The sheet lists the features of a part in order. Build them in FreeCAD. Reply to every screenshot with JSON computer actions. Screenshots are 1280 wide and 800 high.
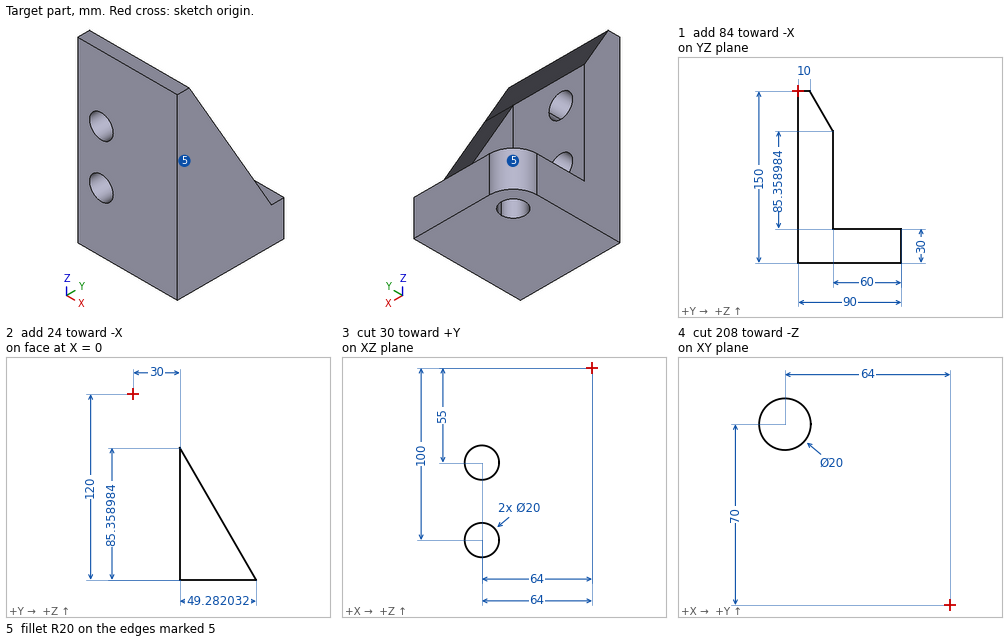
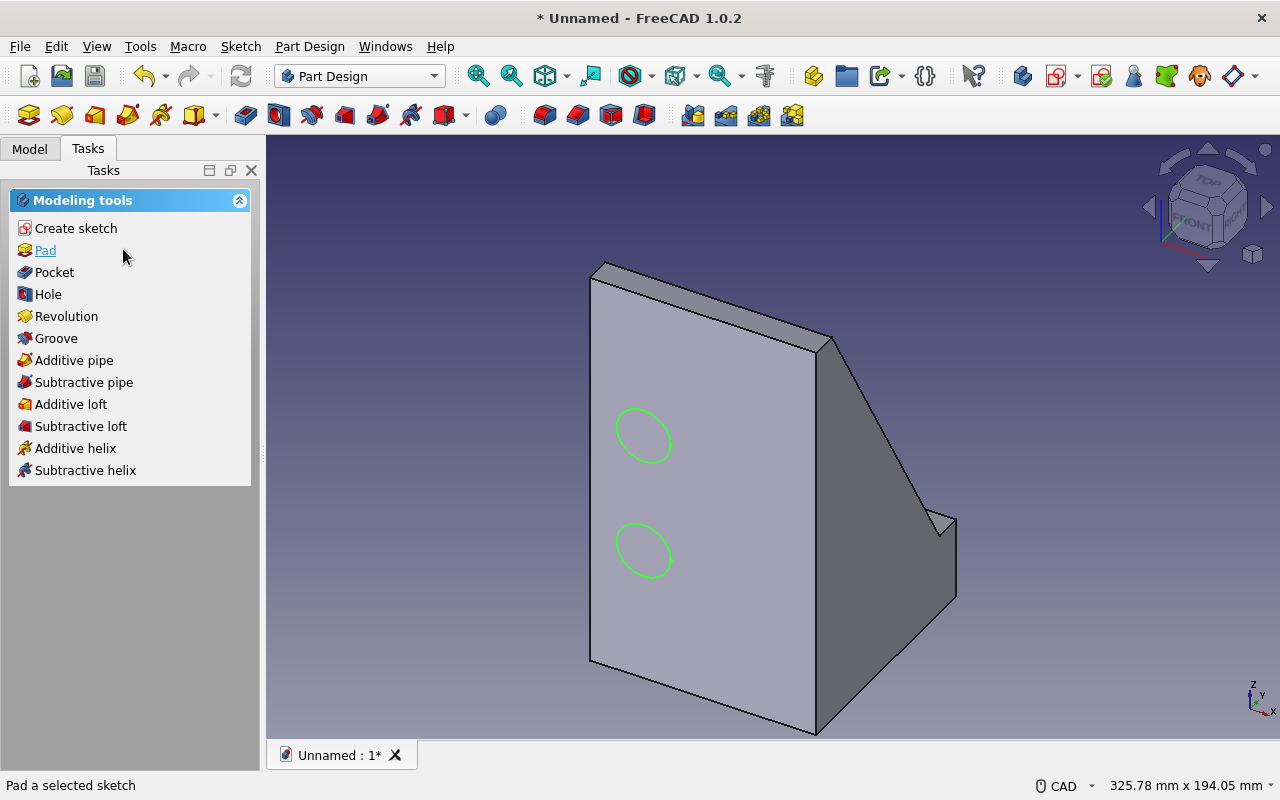
{"action": "left_click", "coordinate": [246, 116]}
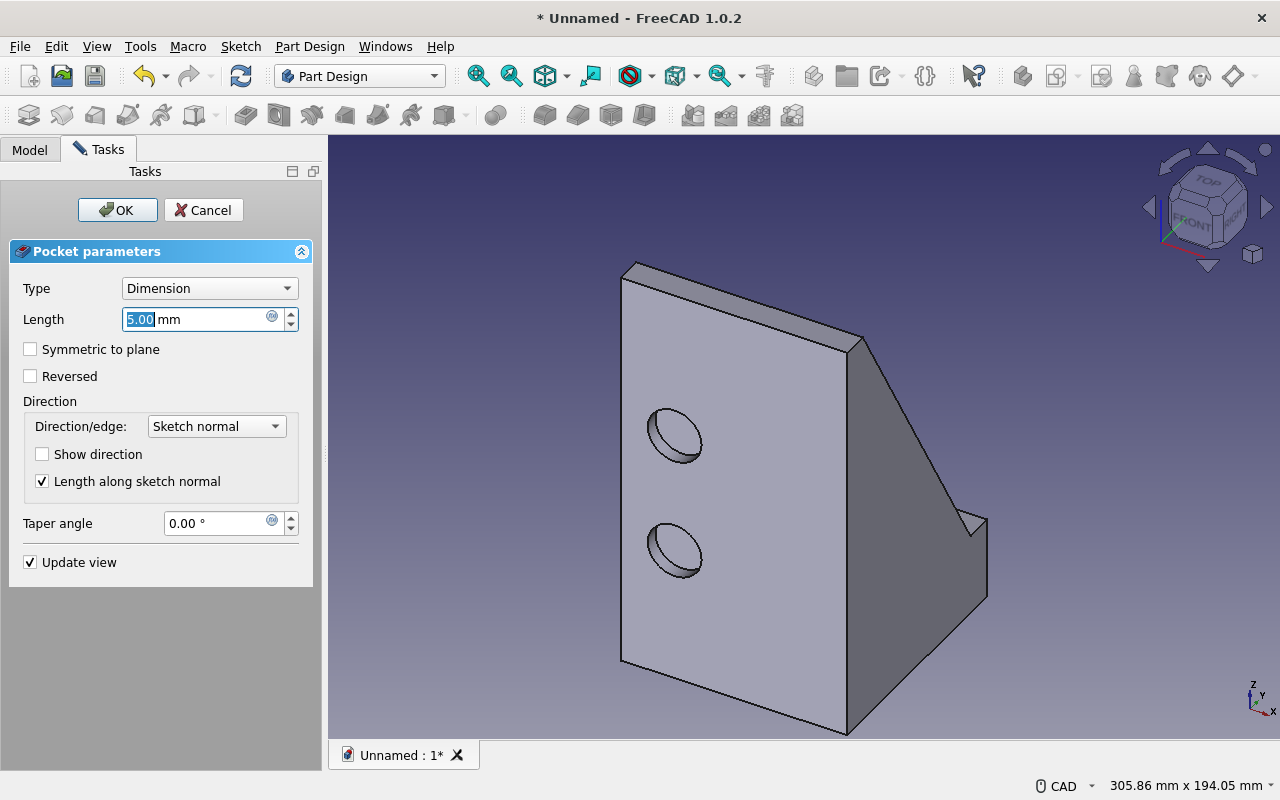
{"action": "type", "text": "30"}
{"action": "key", "text": "Tab"}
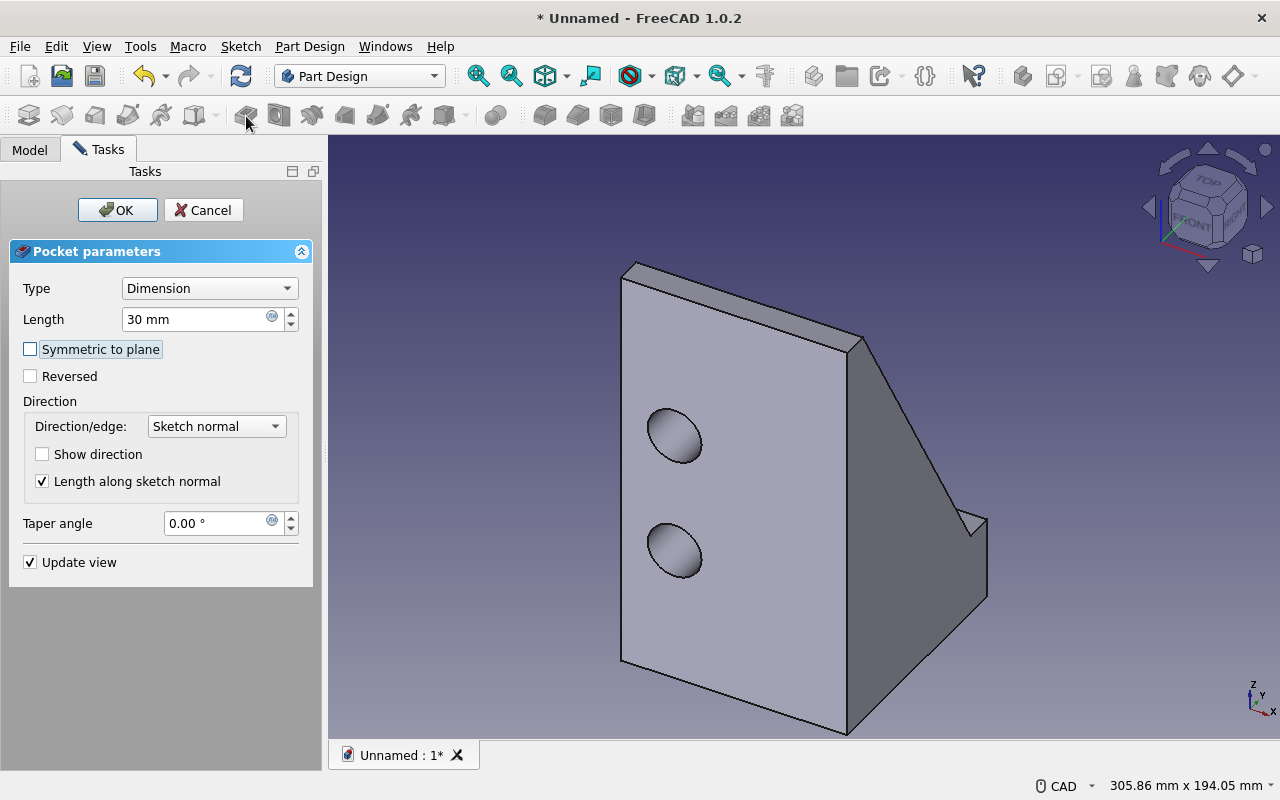
{"action": "left_click", "coordinate": [118, 210]}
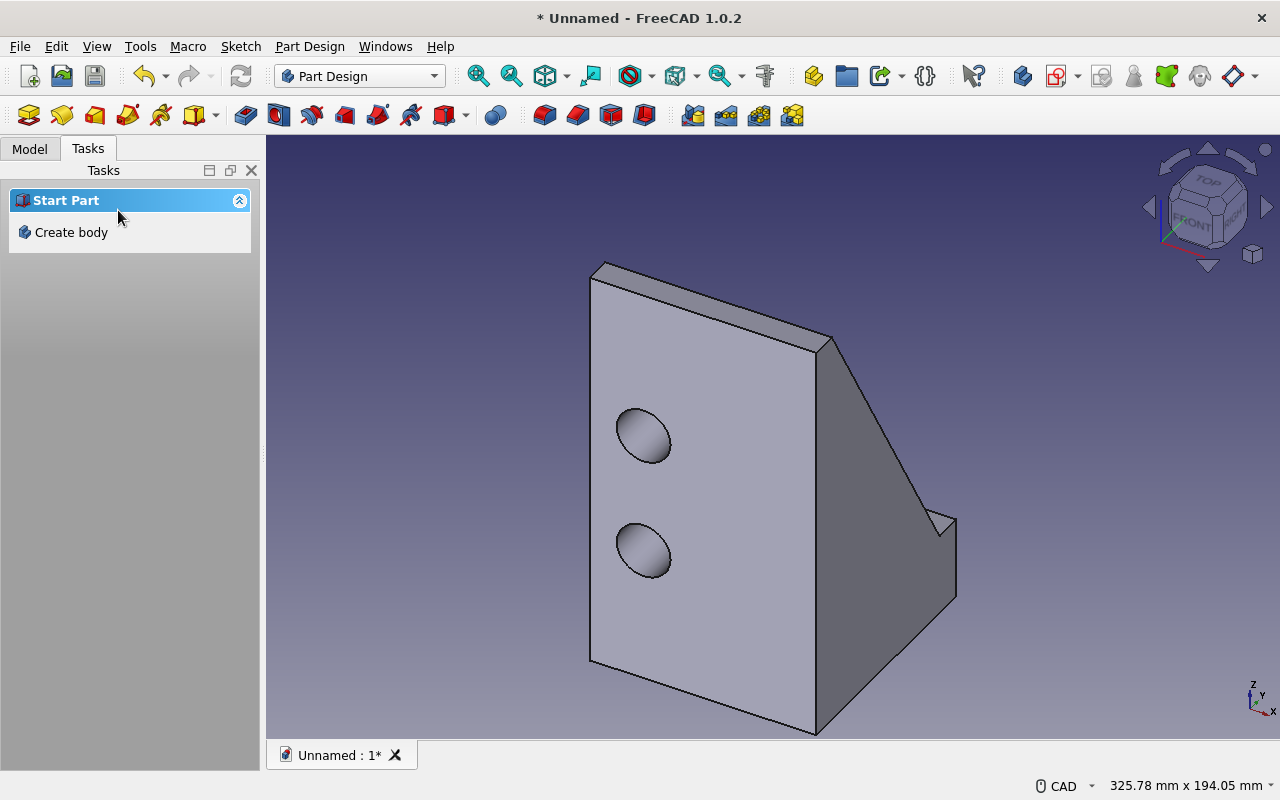
{"action": "left_click", "coordinate": [1056, 76]}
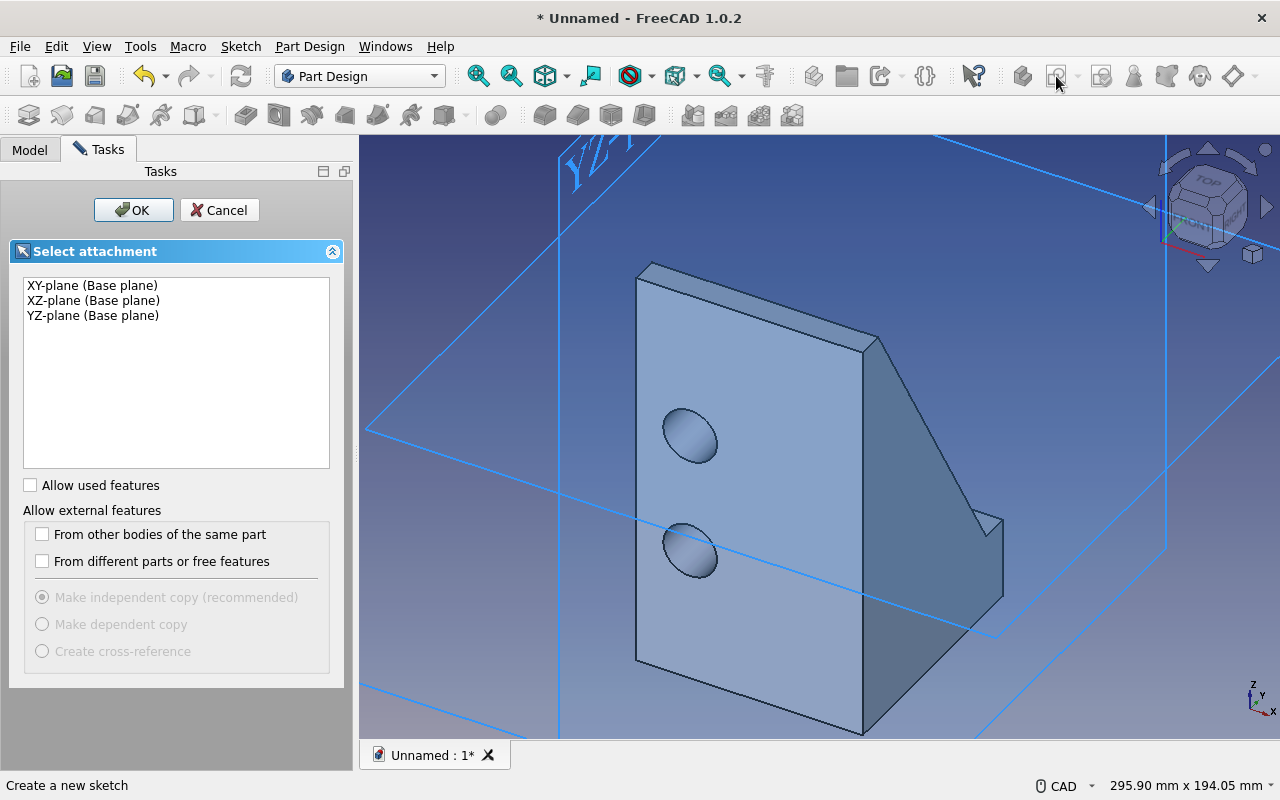
{"action": "left_click", "coordinate": [84, 286]}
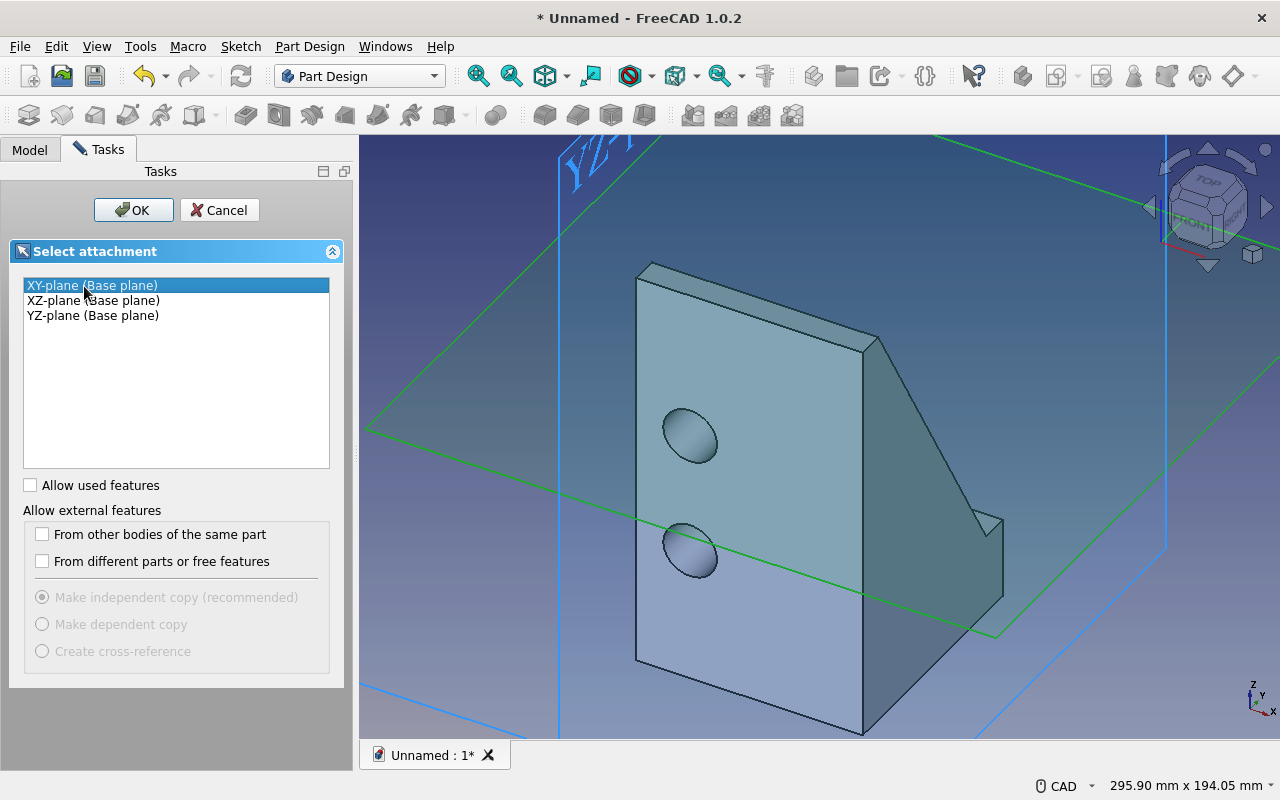
{"action": "left_click", "coordinate": [134, 210]}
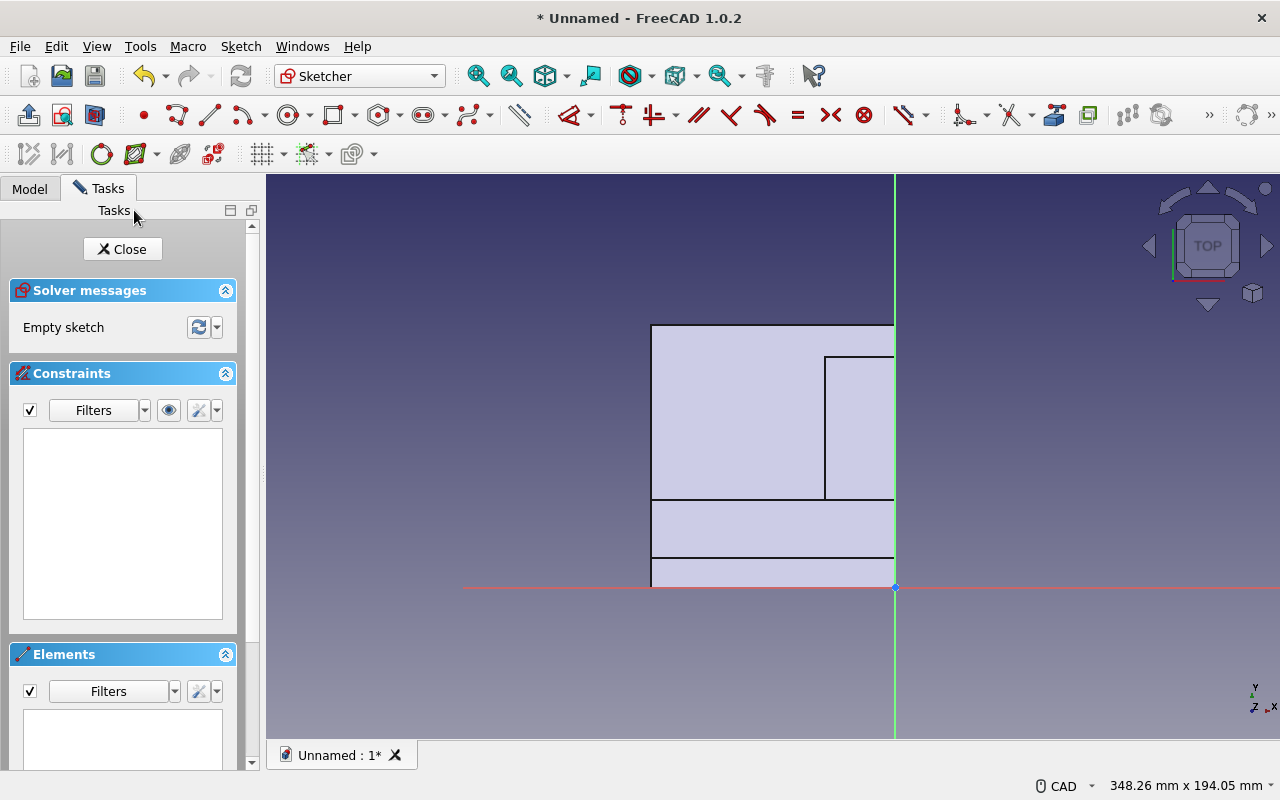
{"action": "scroll", "coordinate": [710, 369], "scroll_direction": "up", "scroll_amount": 9}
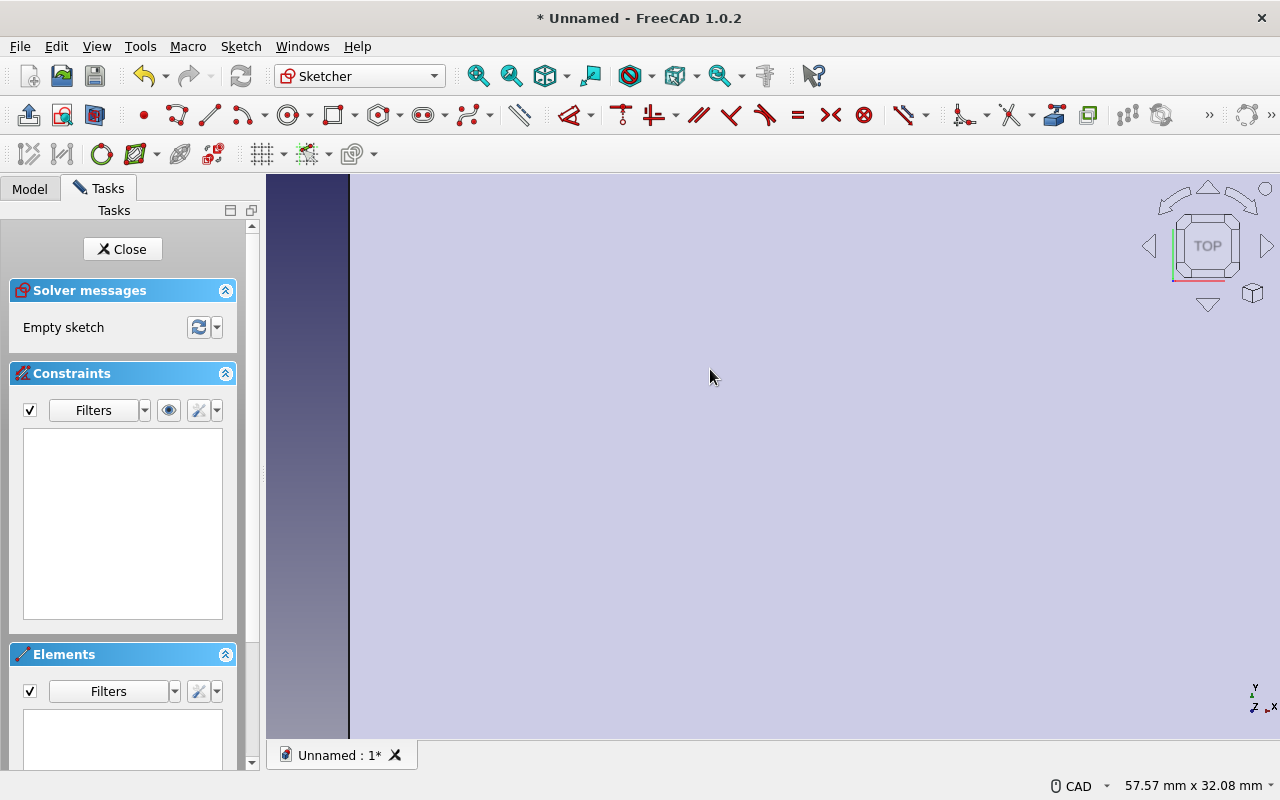
{"action": "left_click", "coordinate": [288, 116]}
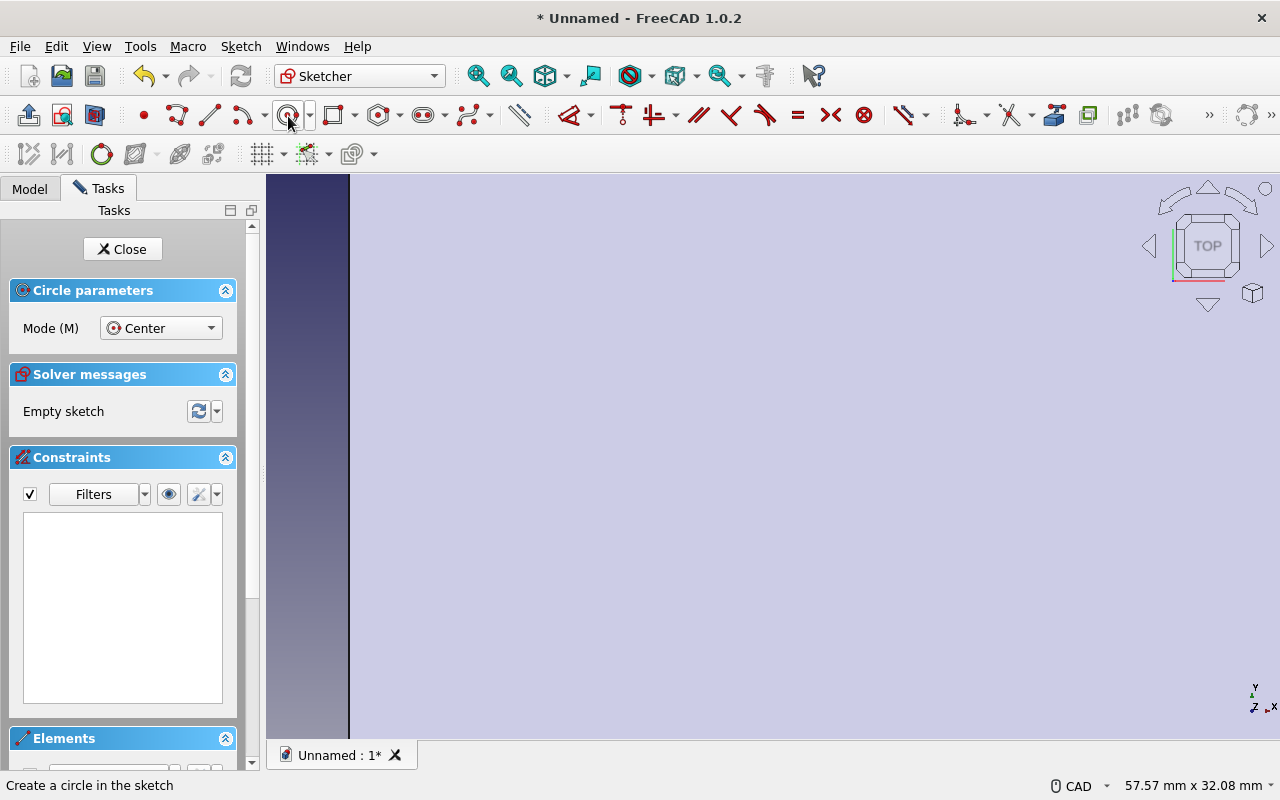
{"action": "left_click", "coordinate": [701, 456]}
{"action": "left_click", "coordinate": [826, 332]}
{"action": "key", "text": "Escape"}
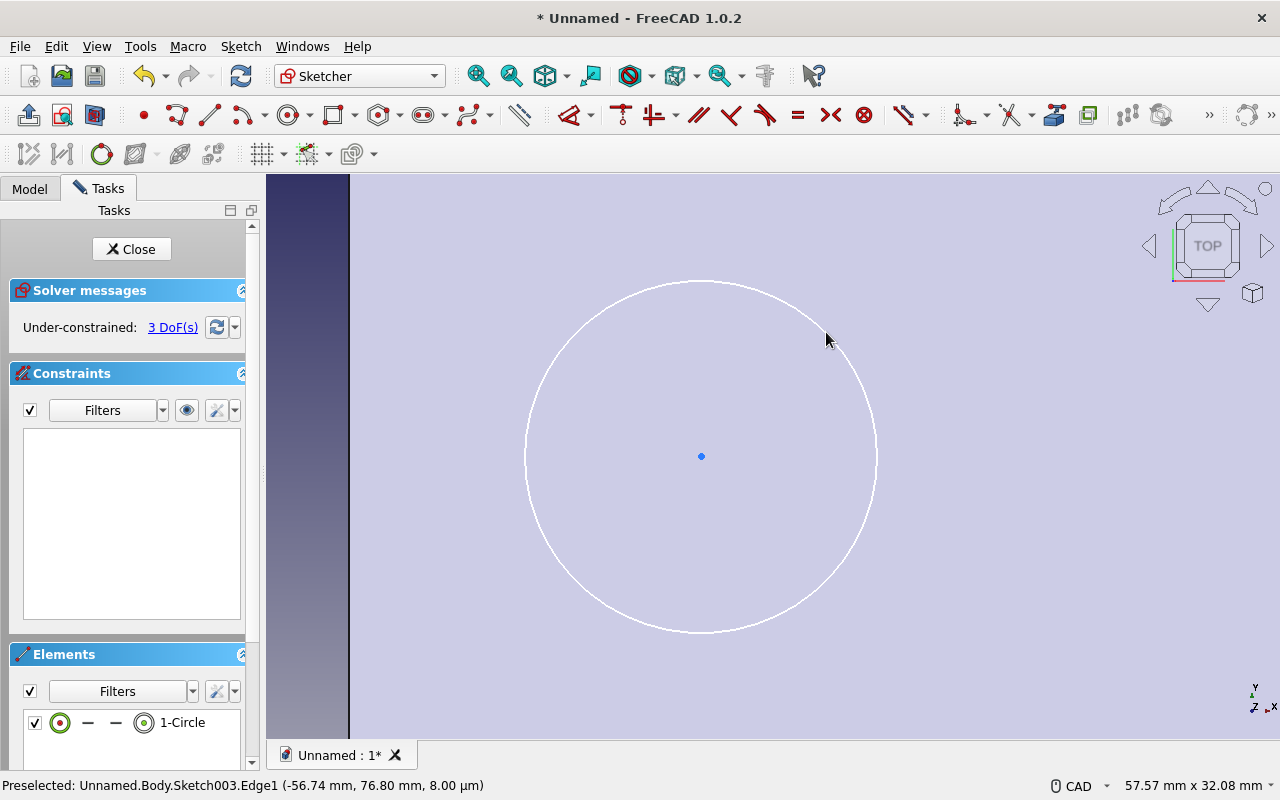
{"action": "left_click", "coordinate": [568, 116]}